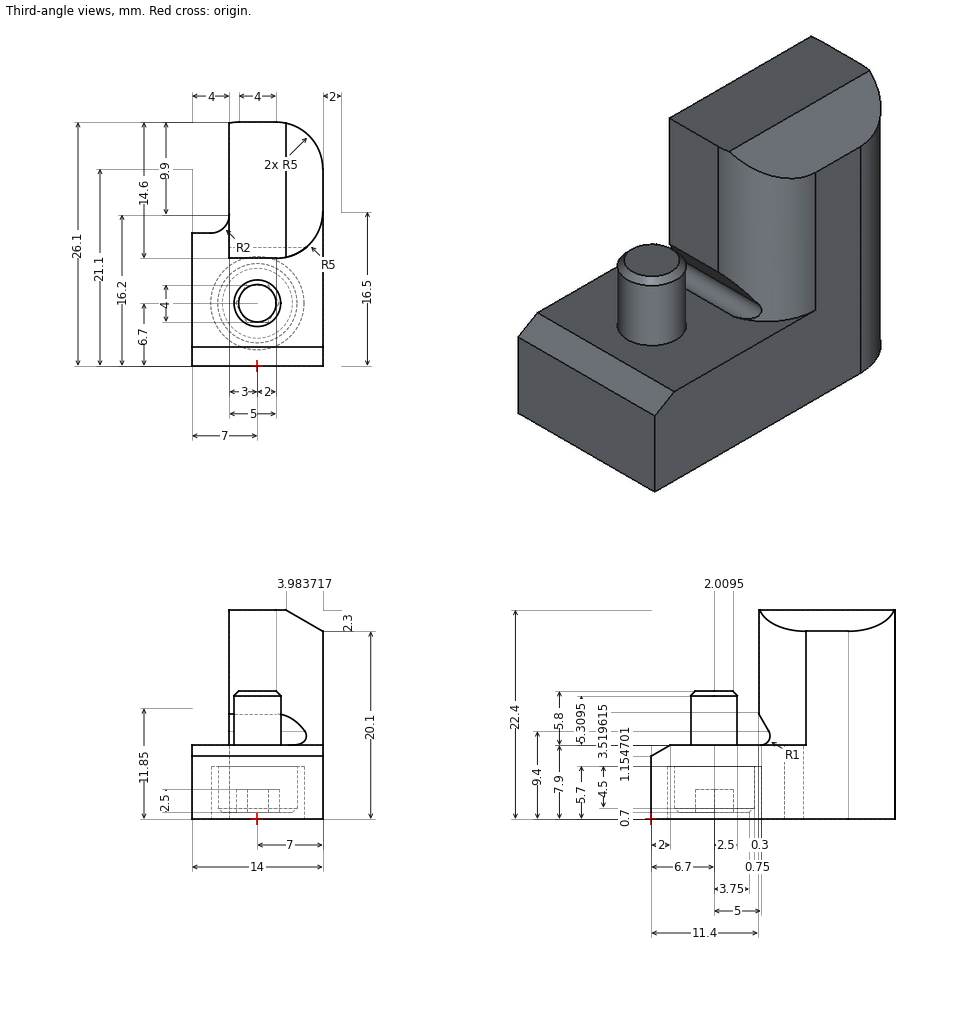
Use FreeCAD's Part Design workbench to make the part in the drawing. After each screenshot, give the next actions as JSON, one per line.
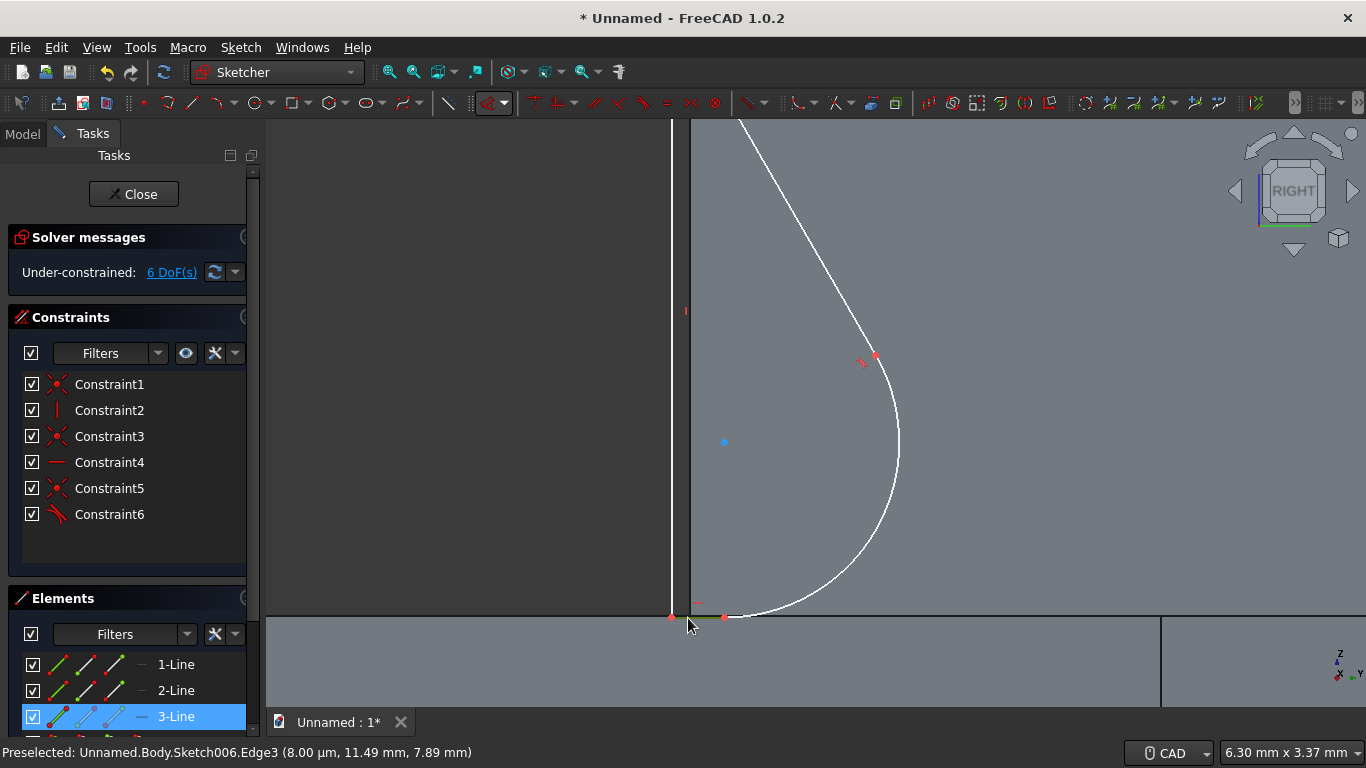
{"action": "left_click", "coordinate": [827, 584]}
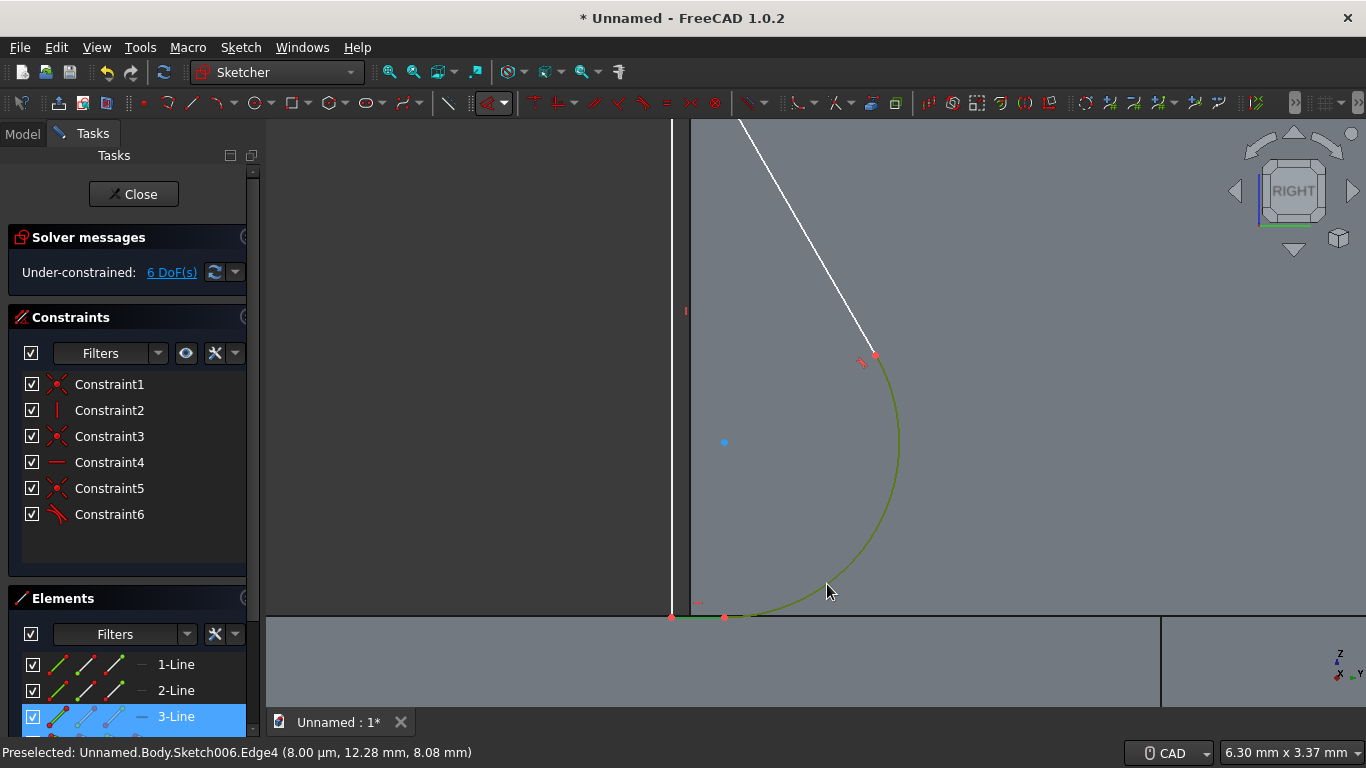
{"action": "left_click", "coordinate": [644, 104]}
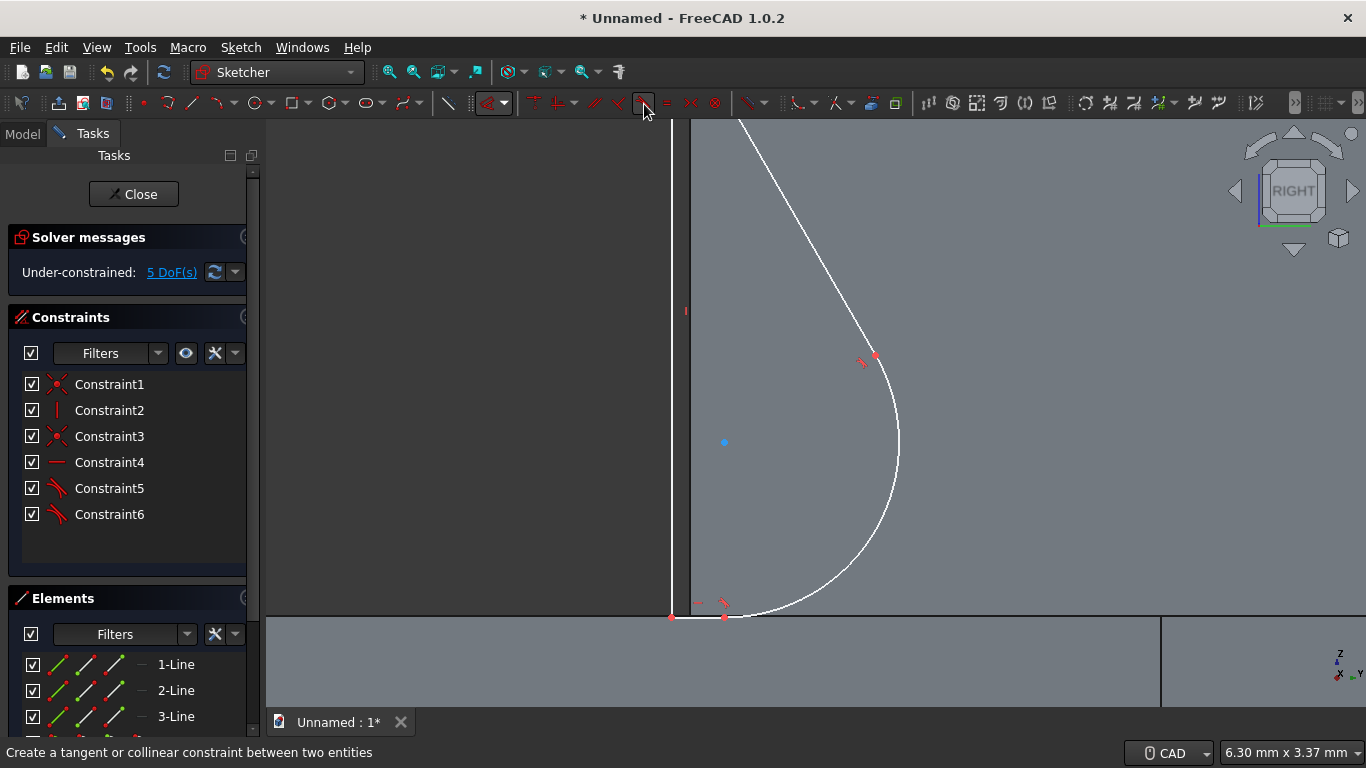
{"action": "left_click", "coordinate": [827, 584]}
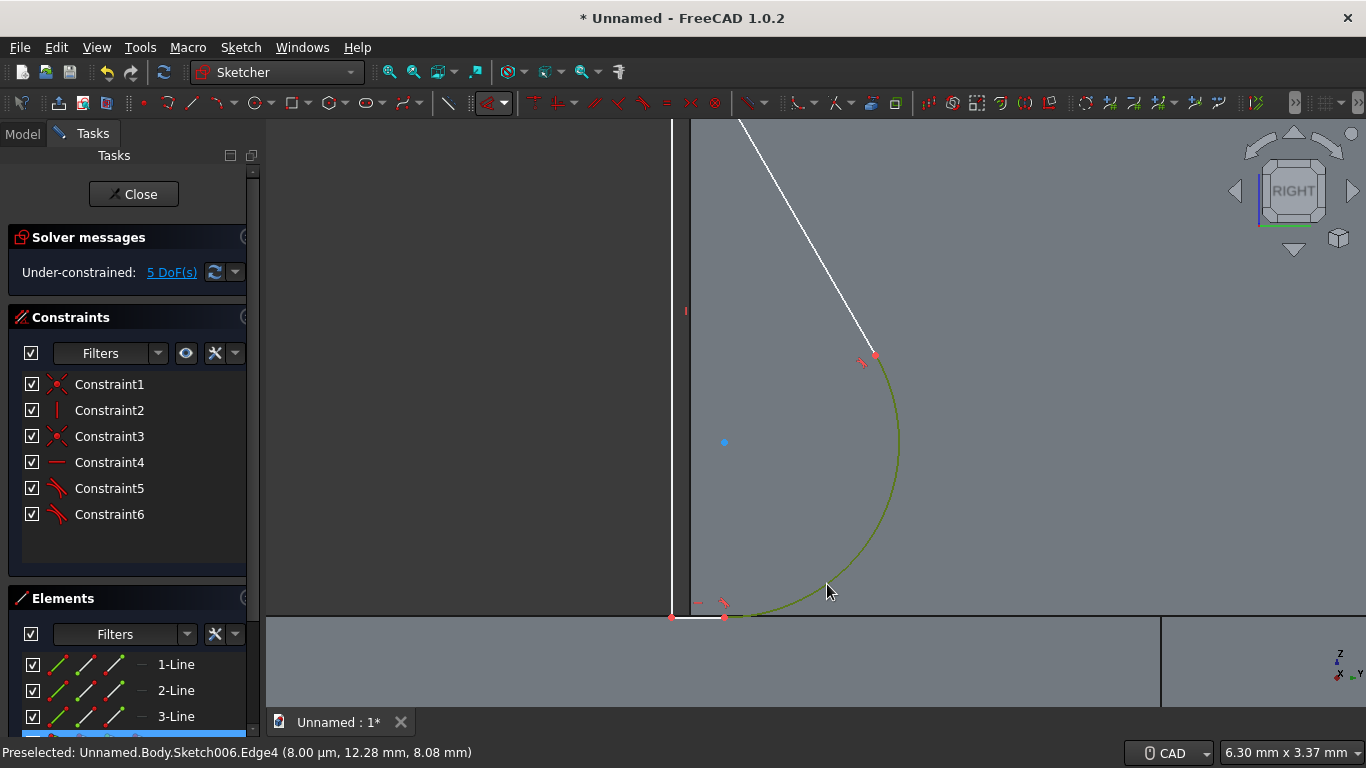
{"action": "left_click", "coordinate": [506, 104]}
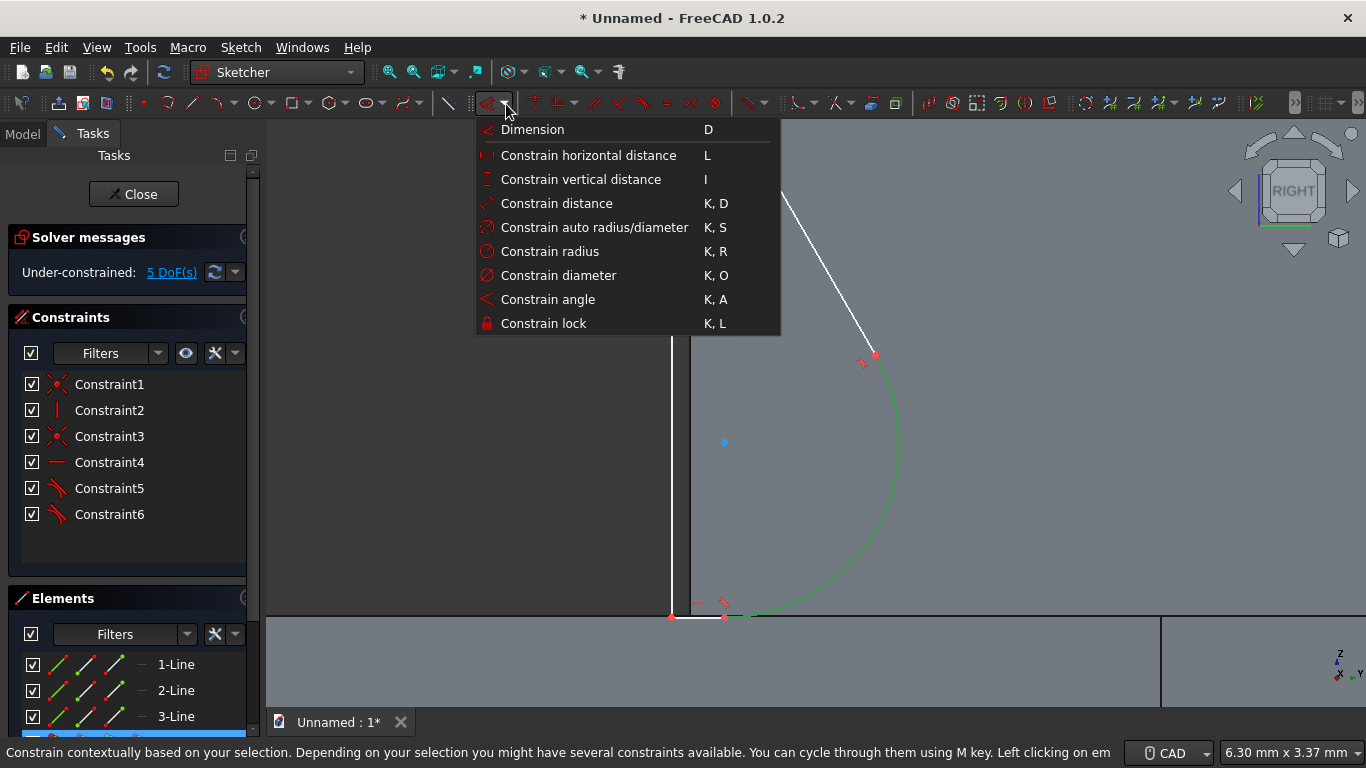
{"action": "left_click", "coordinate": [628, 251]}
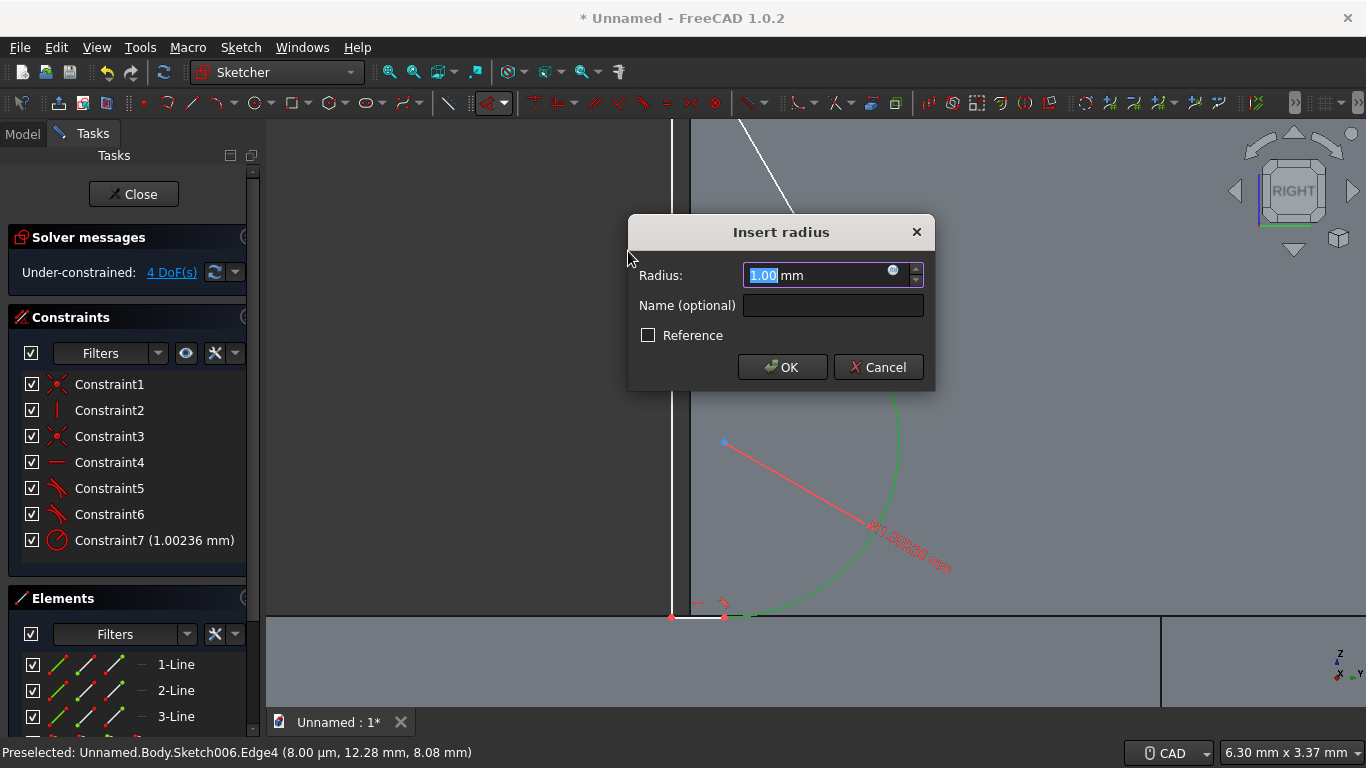
{"action": "type", "text": "1"}
{"action": "key", "text": "Return"}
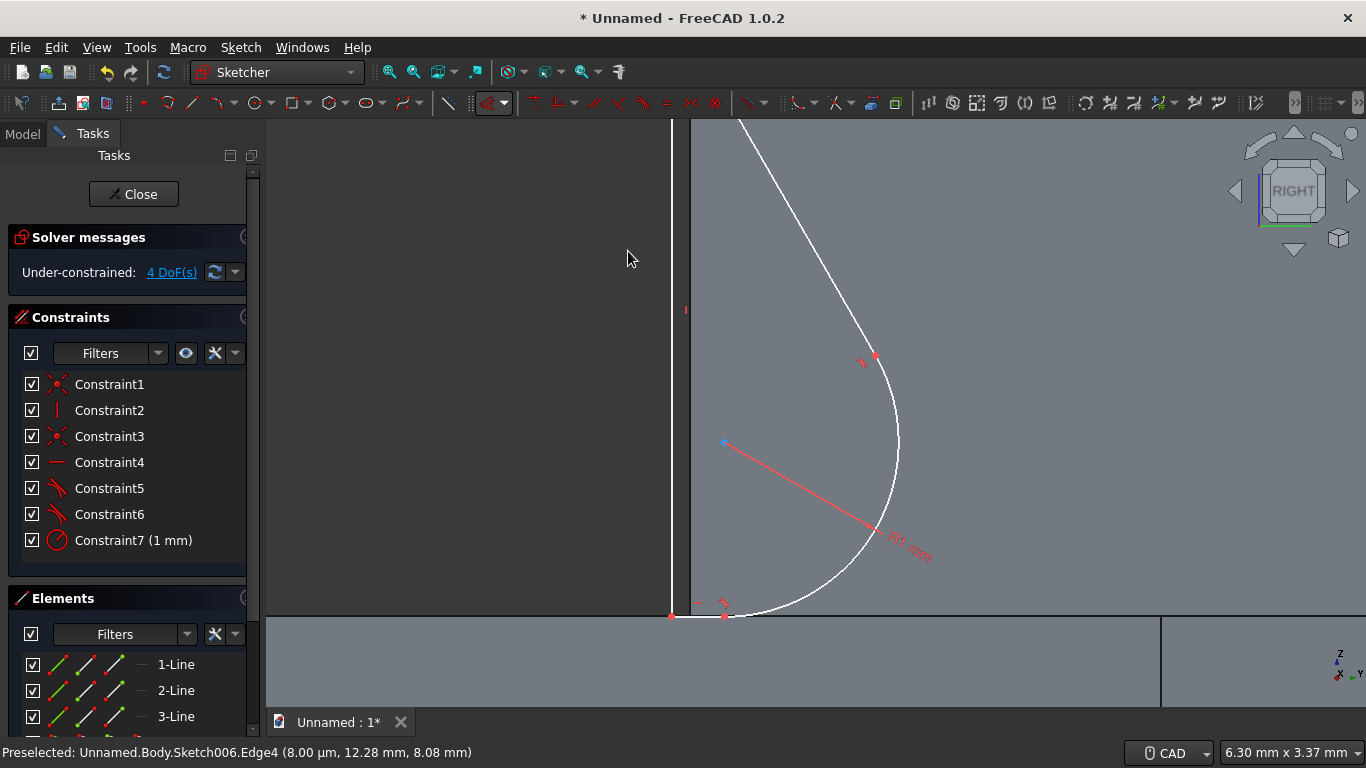
{"action": "left_click", "coordinate": [688, 617]}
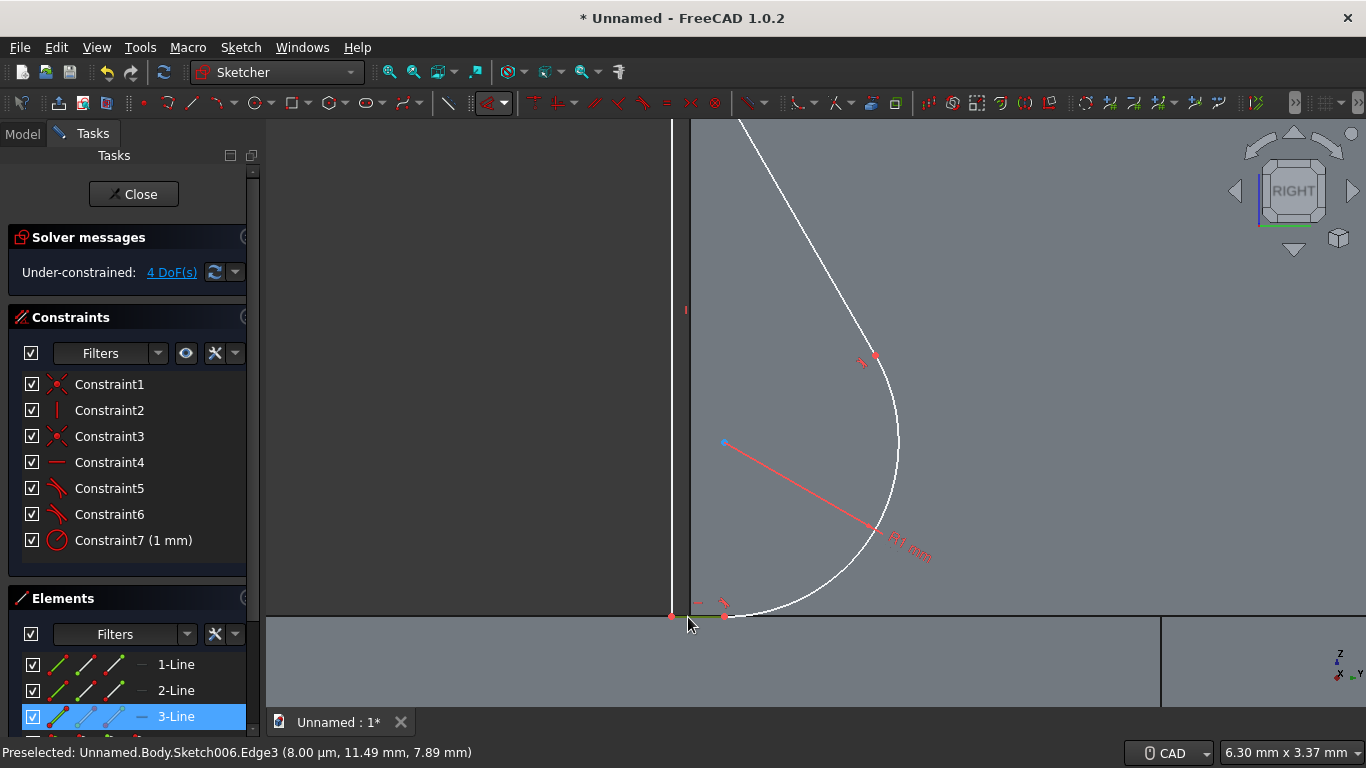
{"action": "left_click", "coordinate": [506, 104]}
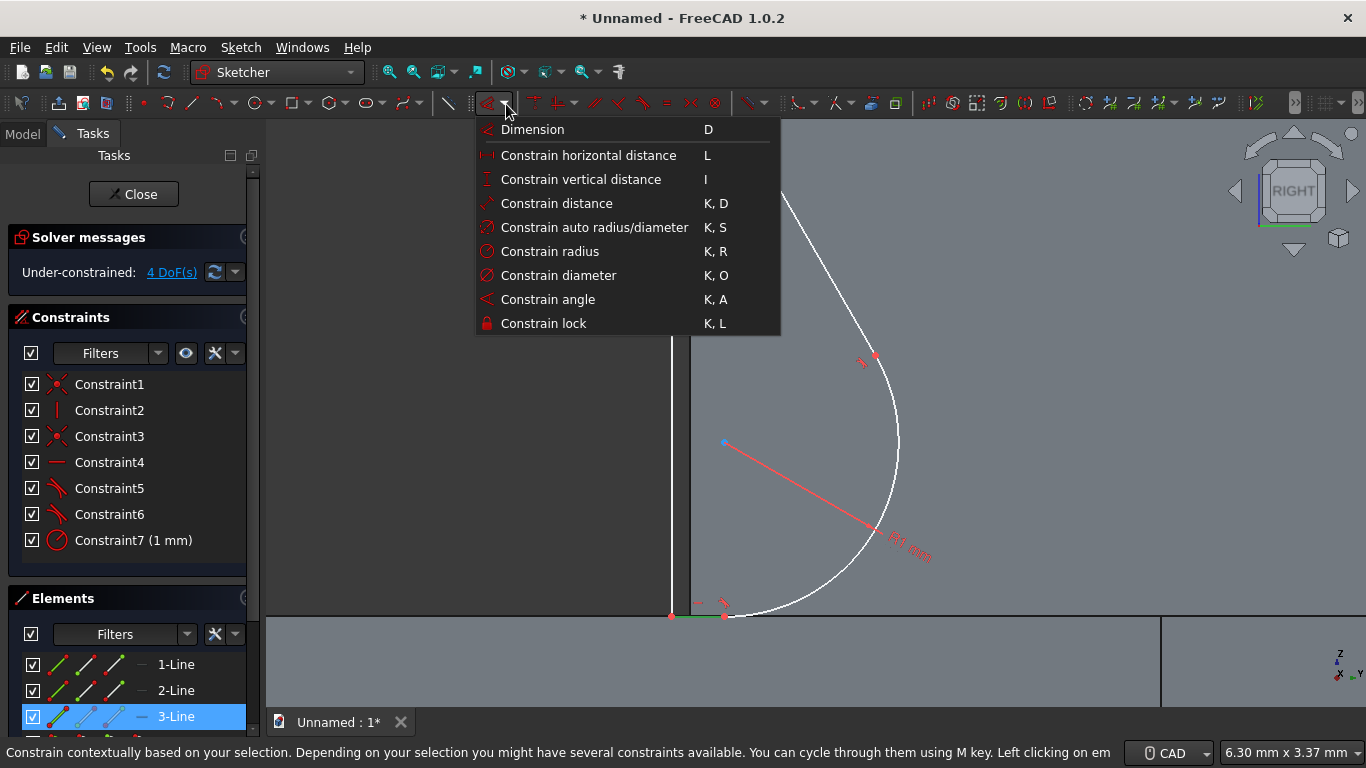
{"action": "left_click", "coordinate": [628, 155]}